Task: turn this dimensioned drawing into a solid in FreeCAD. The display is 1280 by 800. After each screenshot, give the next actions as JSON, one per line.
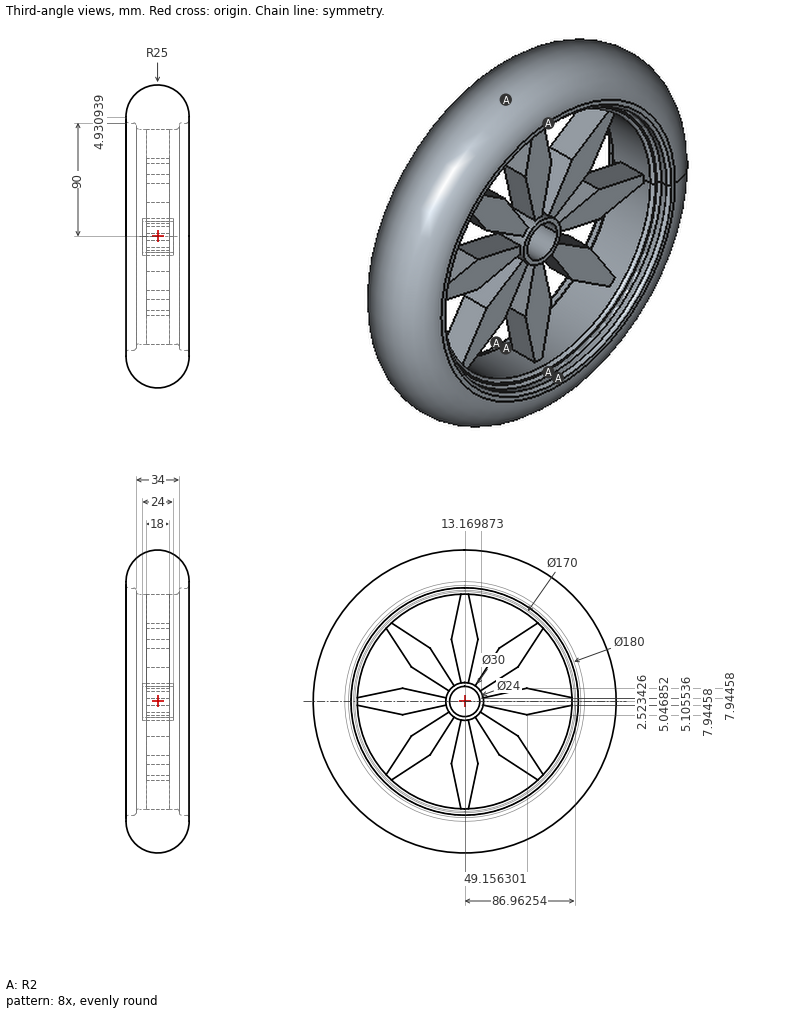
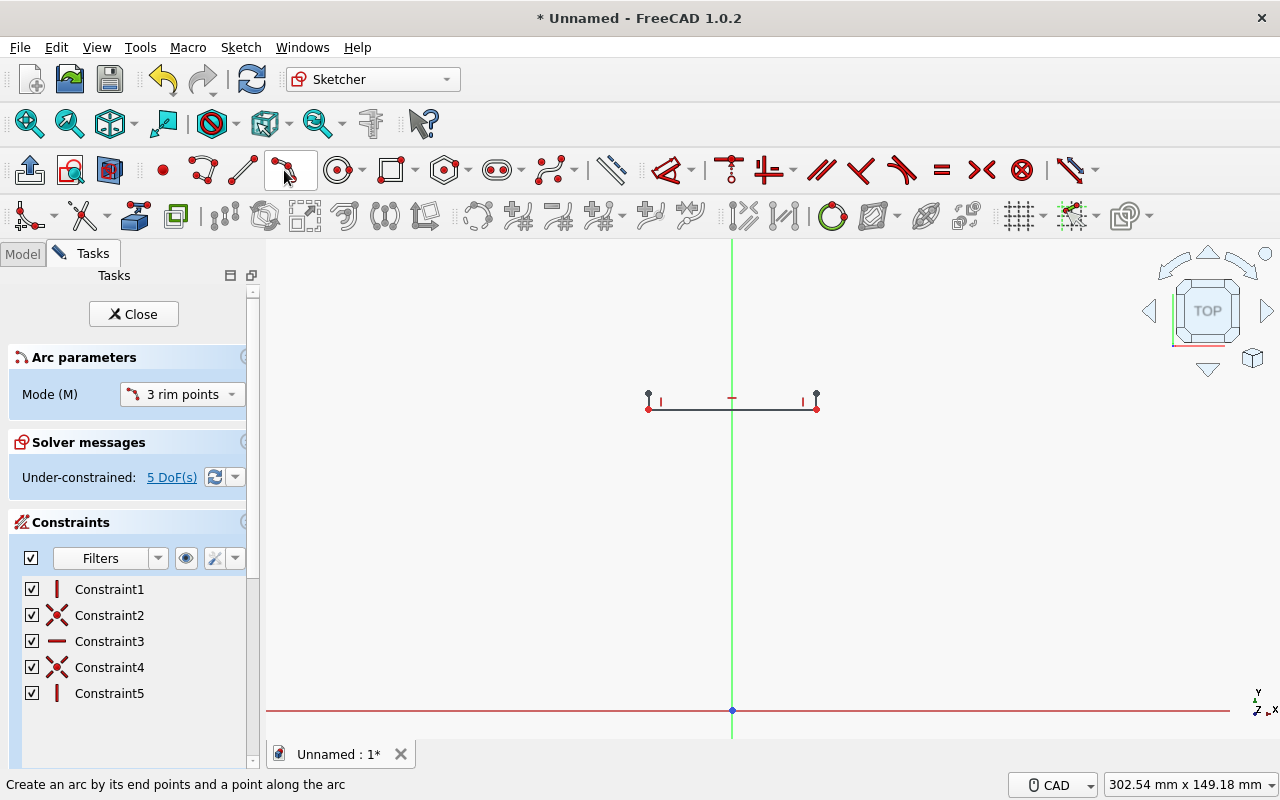
{"action": "scroll", "coordinate": [816, 393], "scroll_direction": "up", "scroll_amount": 4}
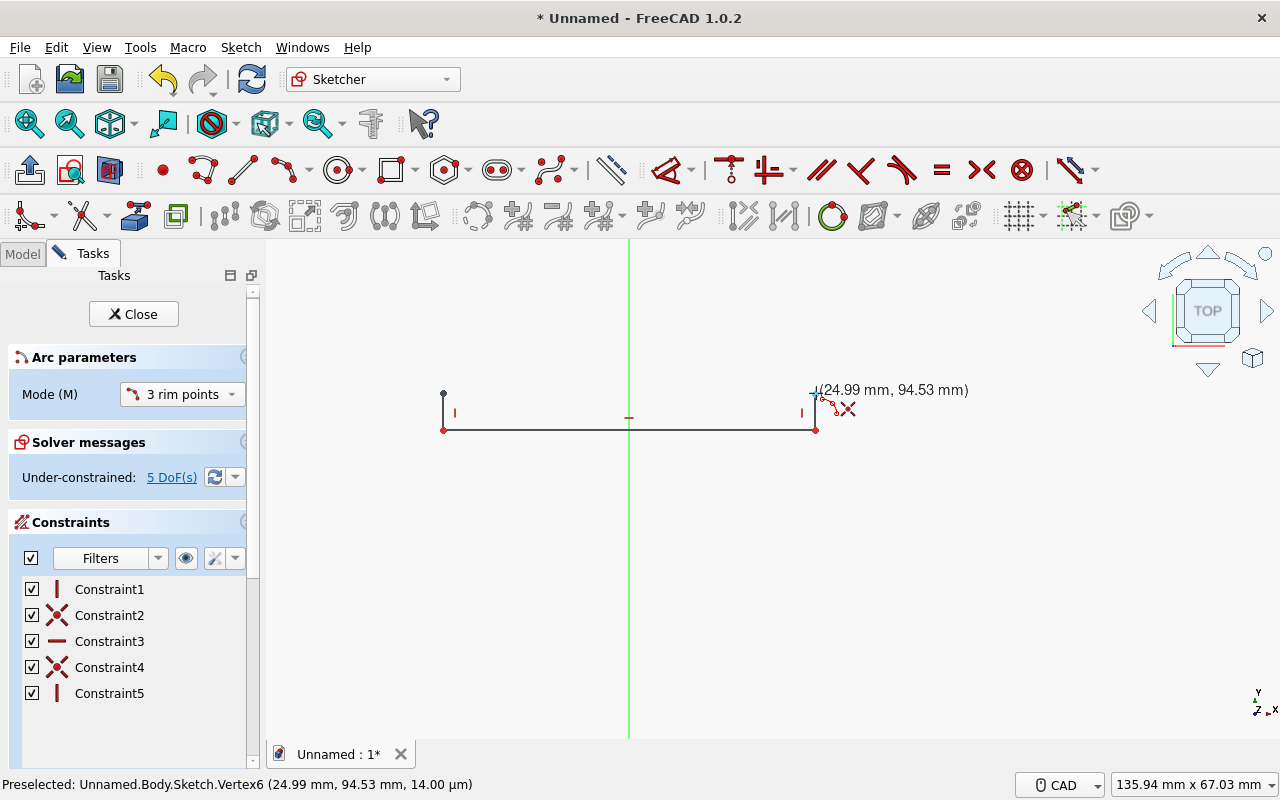
{"action": "left_click", "coordinate": [815, 395]}
{"action": "left_click", "coordinate": [443, 394]}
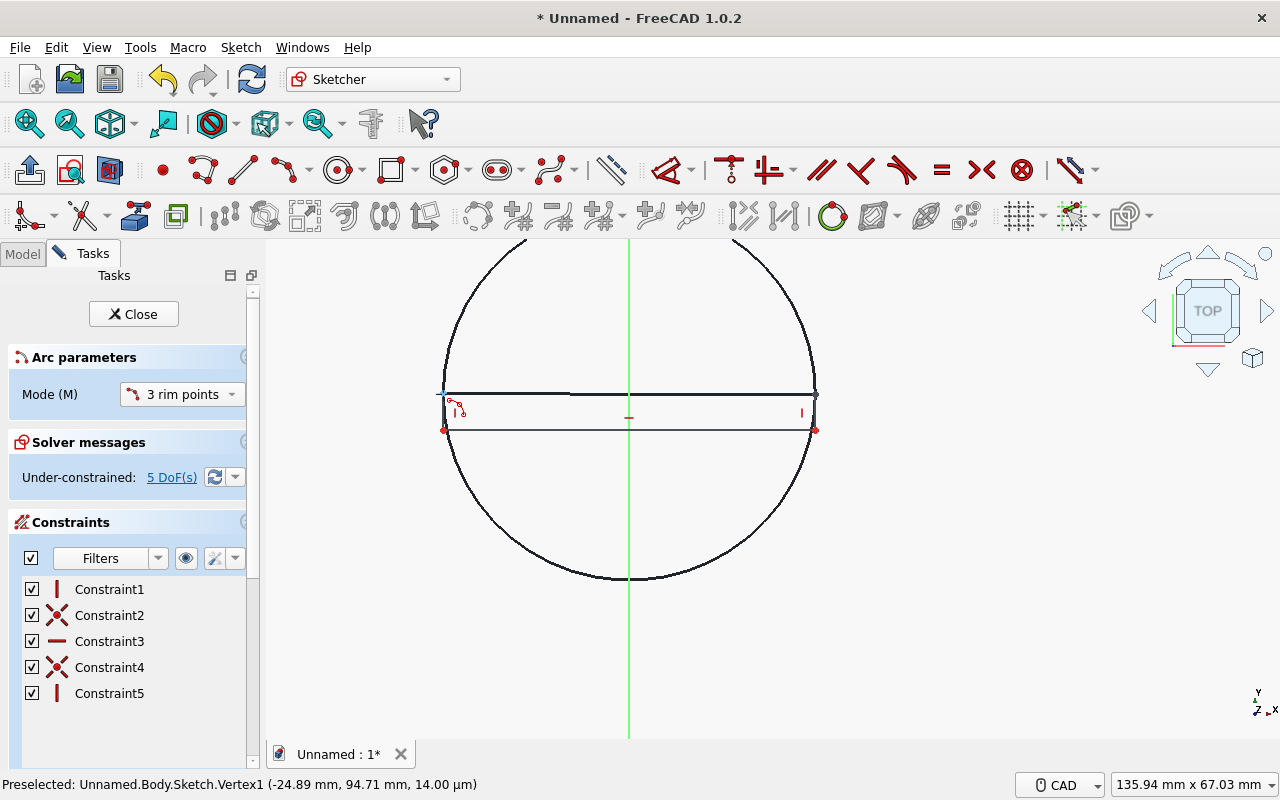
{"action": "scroll", "coordinate": [748, 394], "scroll_direction": "down", "scroll_amount": 5}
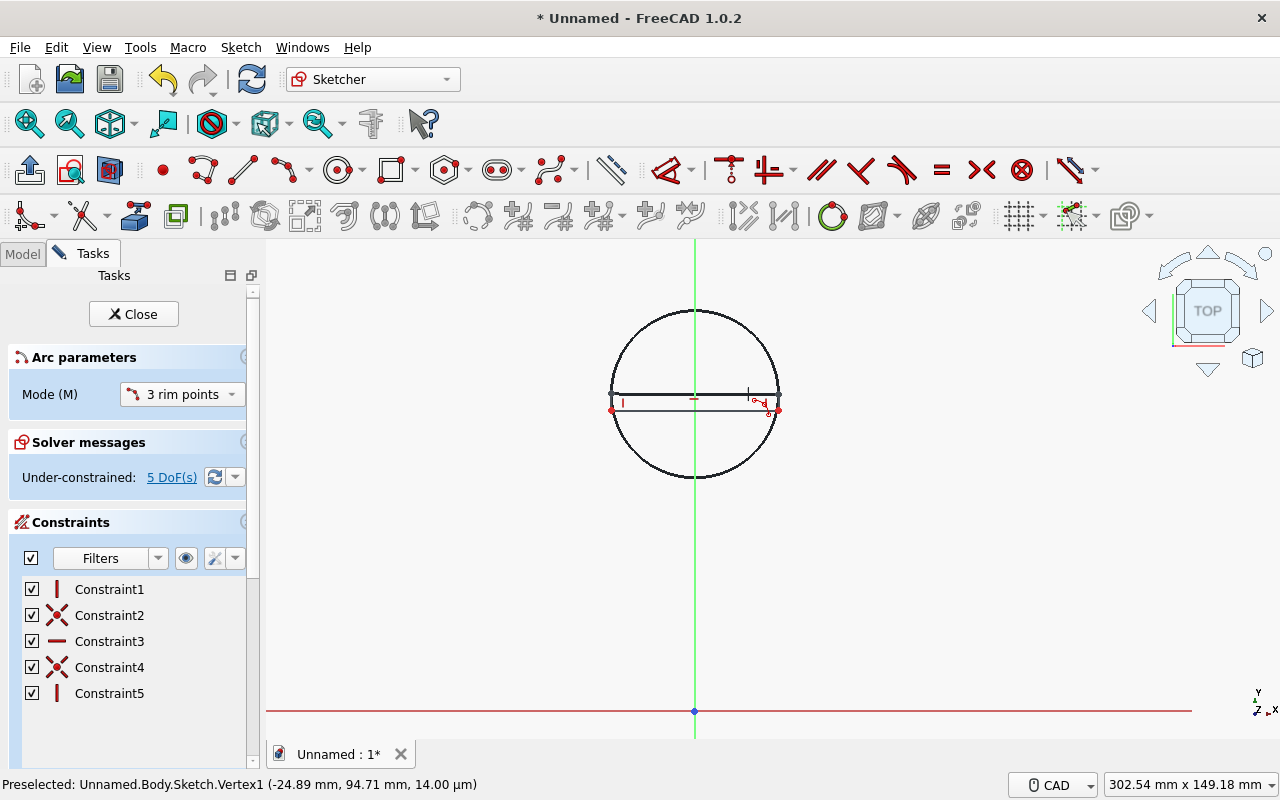
{"action": "left_click", "coordinate": [726, 328]}
{"action": "key", "text": "Escape"}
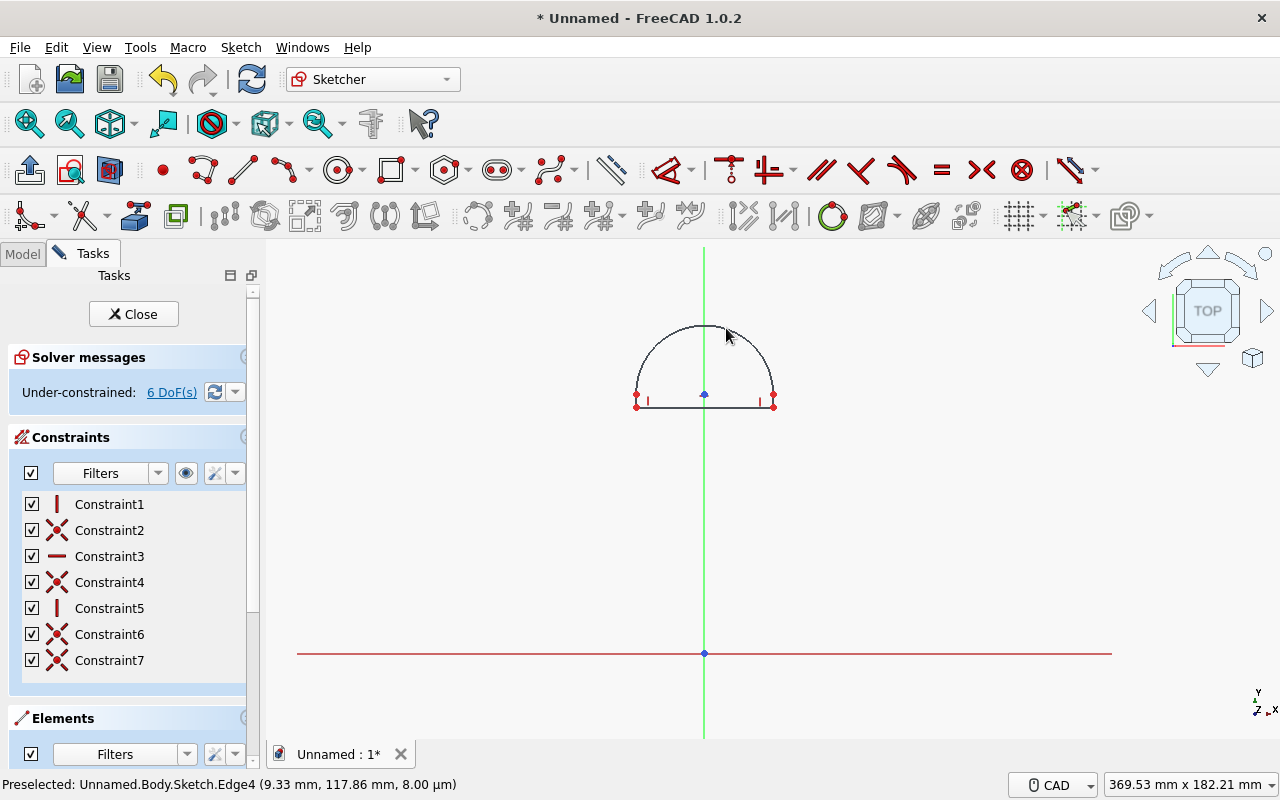
{"action": "scroll", "coordinate": [636, 401], "scroll_direction": "up", "scroll_amount": 4}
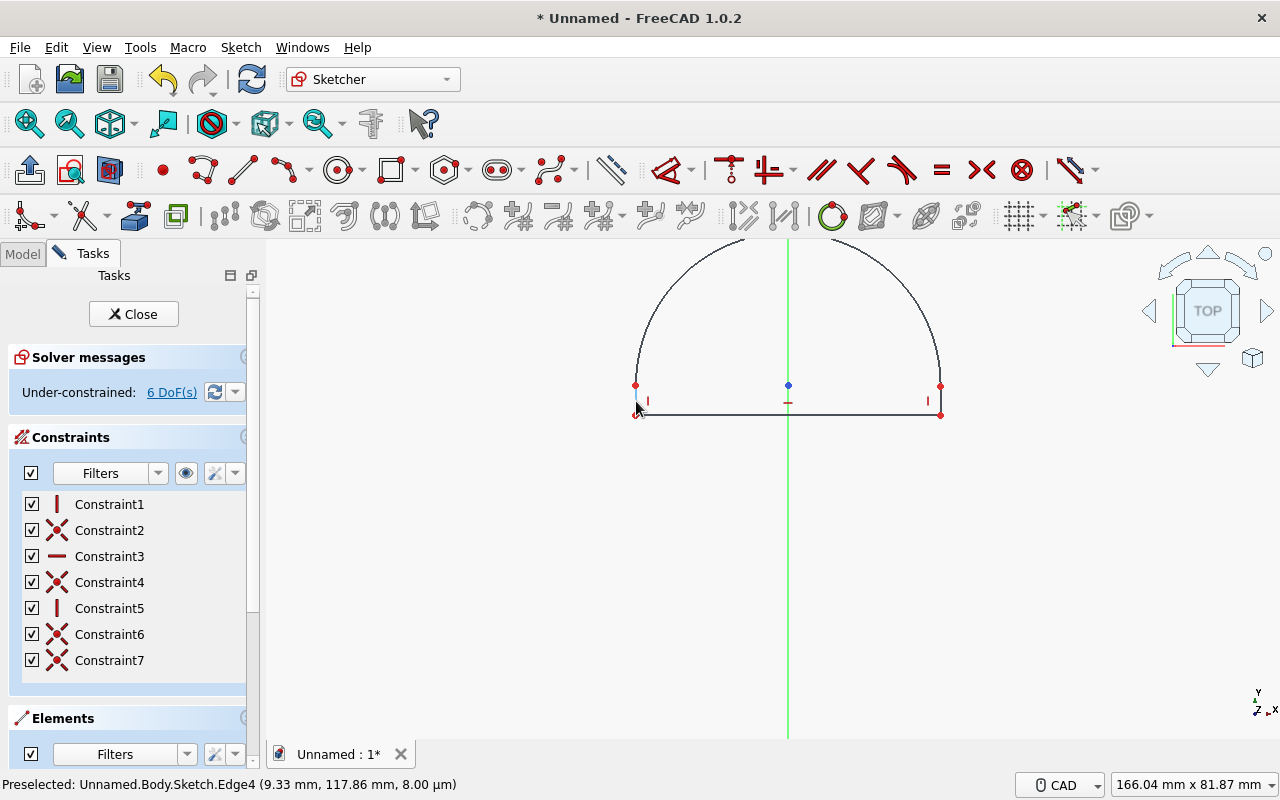
{"action": "left_click", "coordinate": [636, 400]}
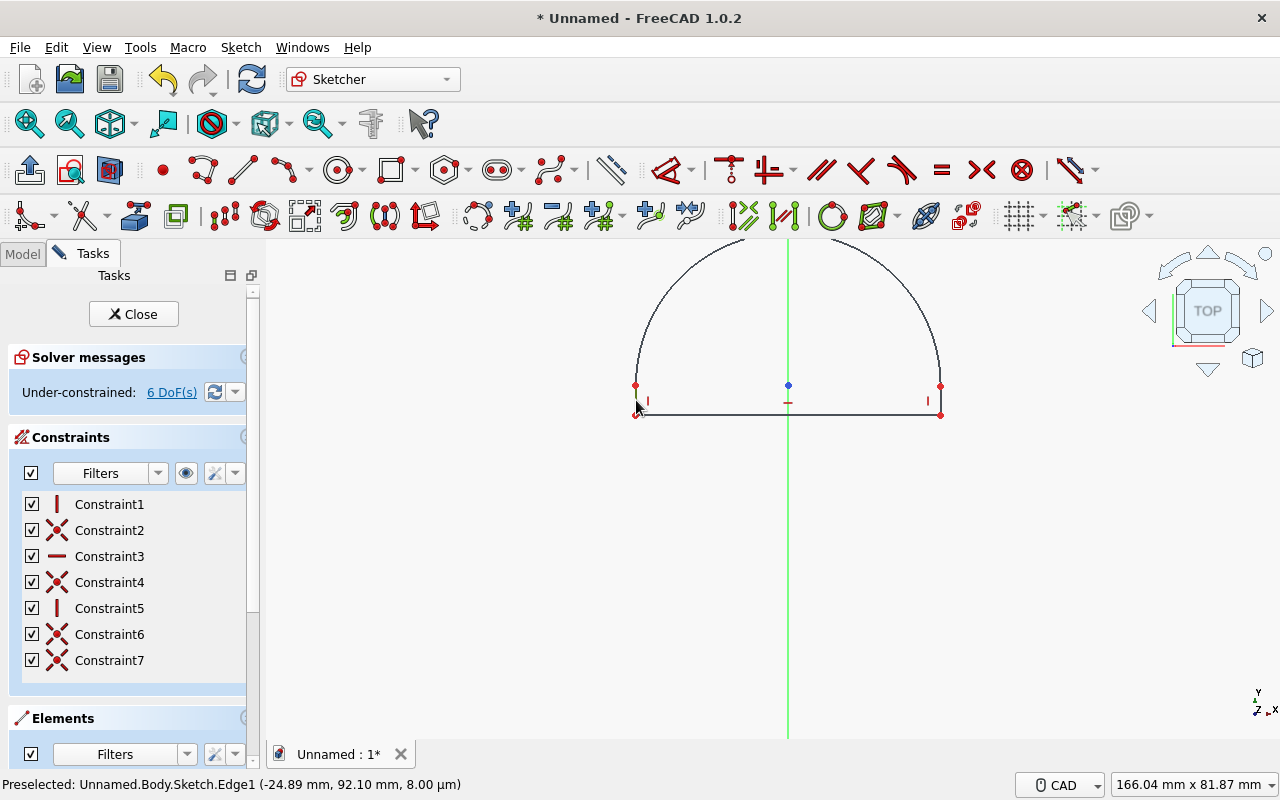
{"action": "left_click", "coordinate": [912, 296]}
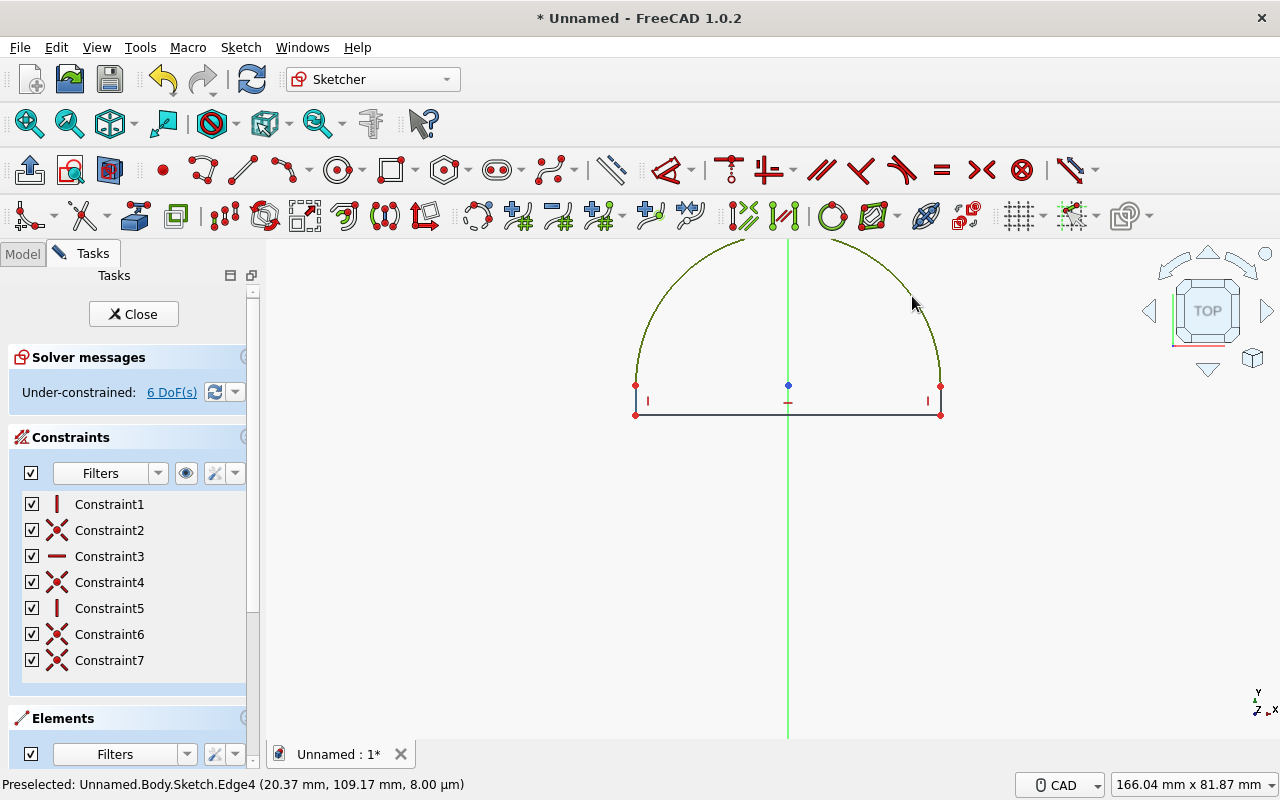
{"action": "left_click", "coordinate": [902, 170]}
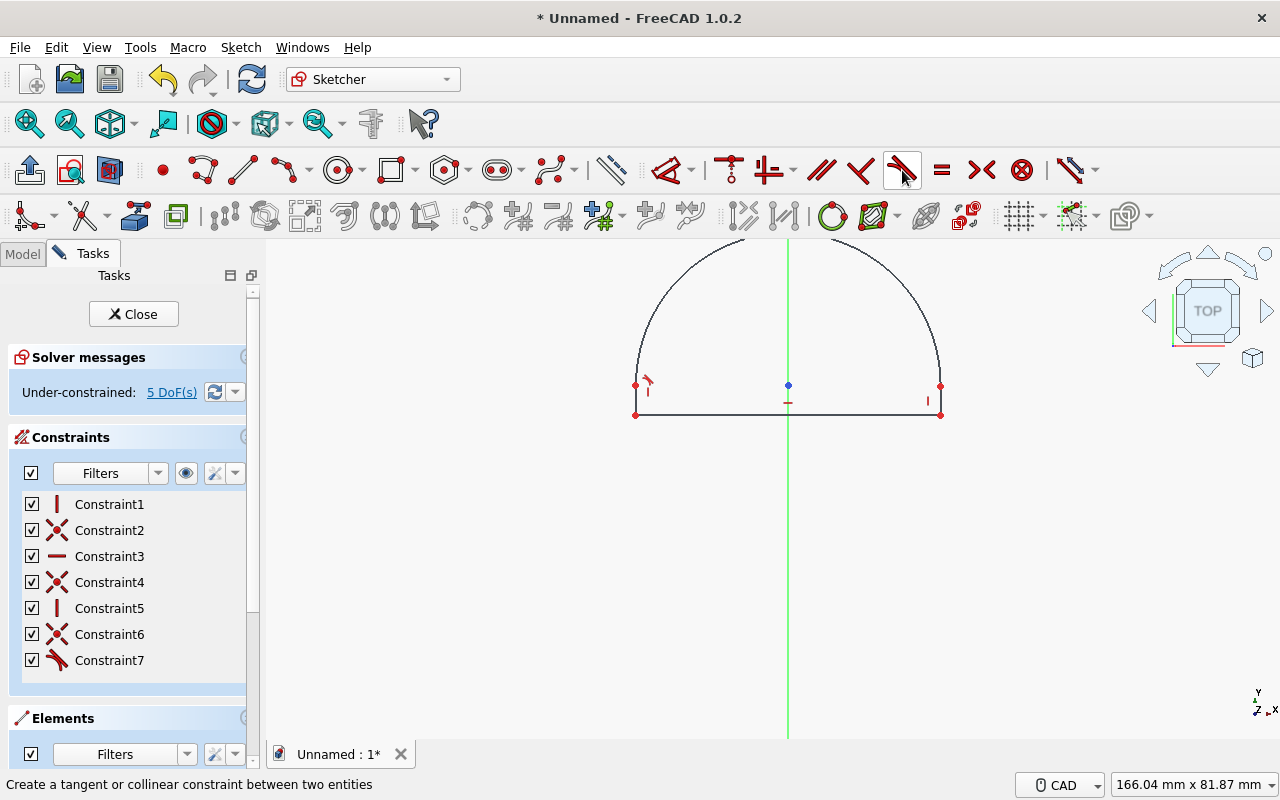
{"action": "left_click", "coordinate": [941, 404]}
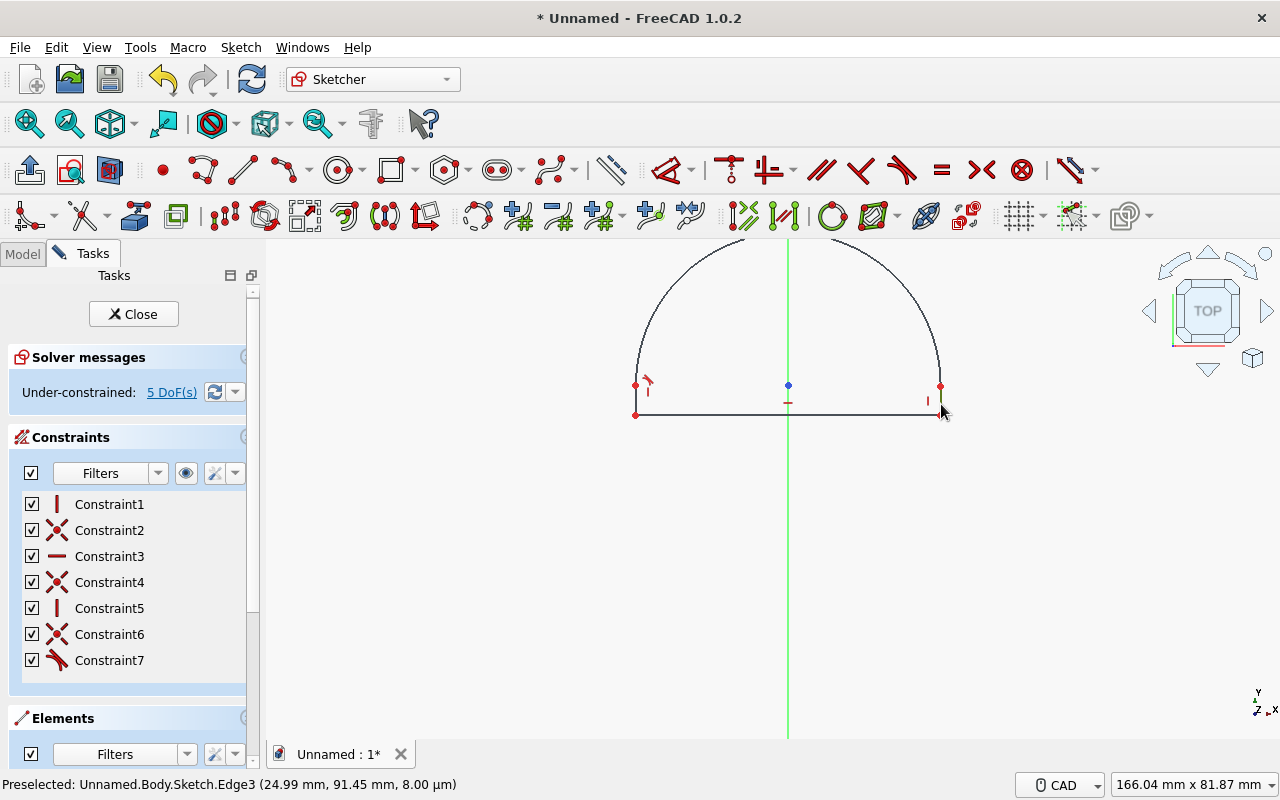
{"action": "left_click", "coordinate": [912, 296]}